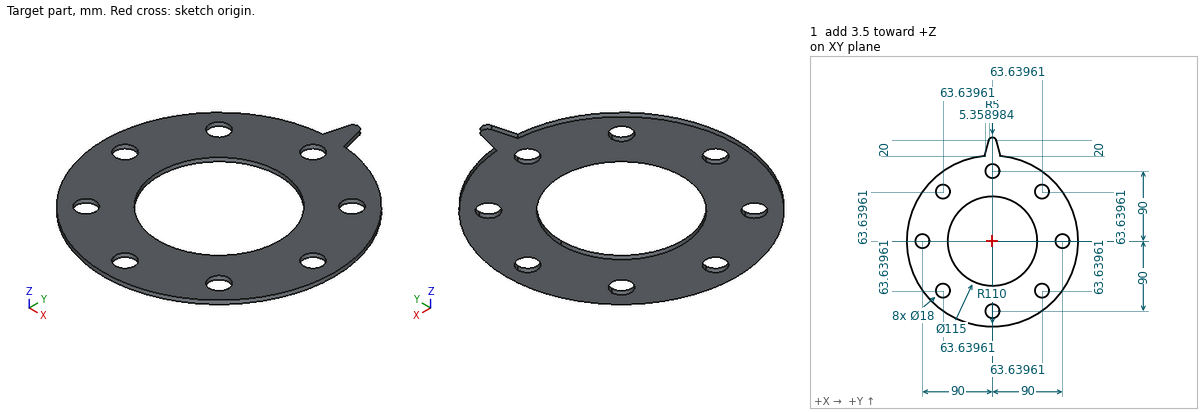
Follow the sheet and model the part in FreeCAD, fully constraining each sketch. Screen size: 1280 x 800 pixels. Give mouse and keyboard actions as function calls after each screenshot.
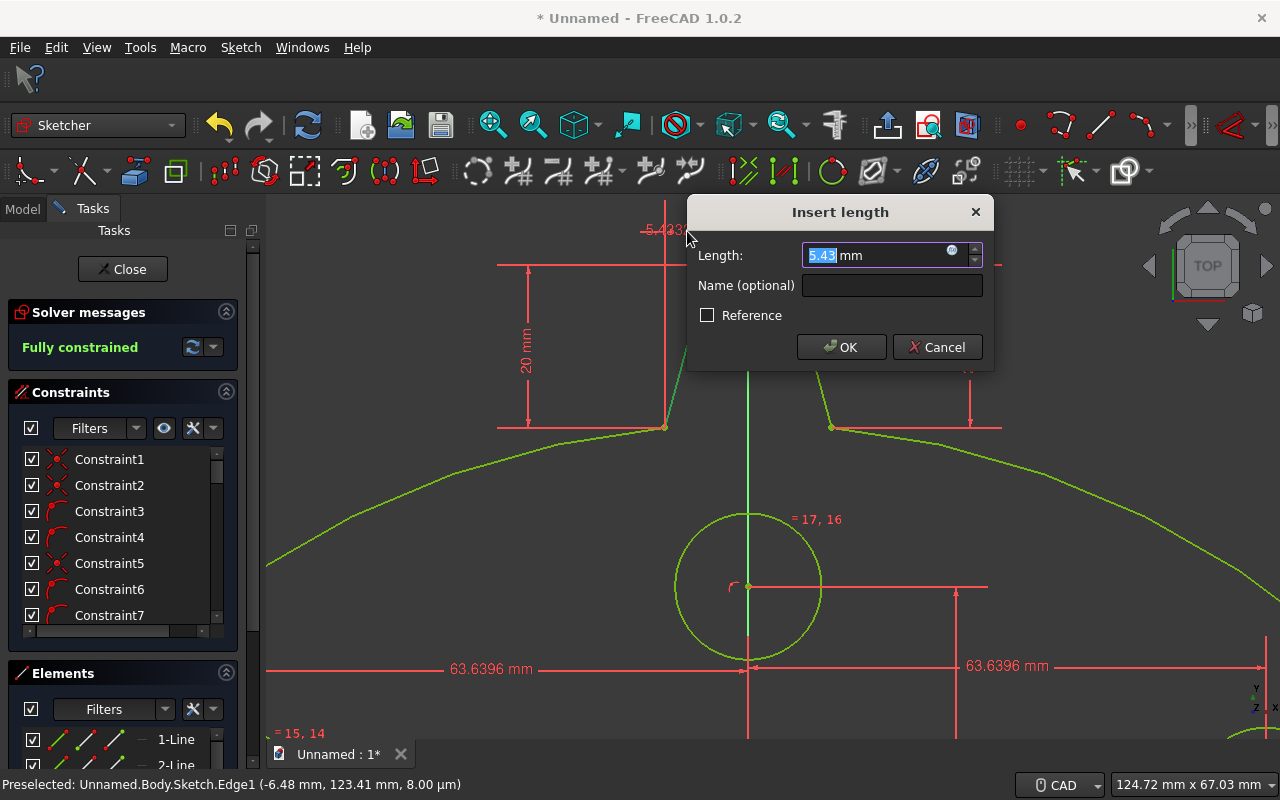
text(5.358984)
key(Return)
key(Escape)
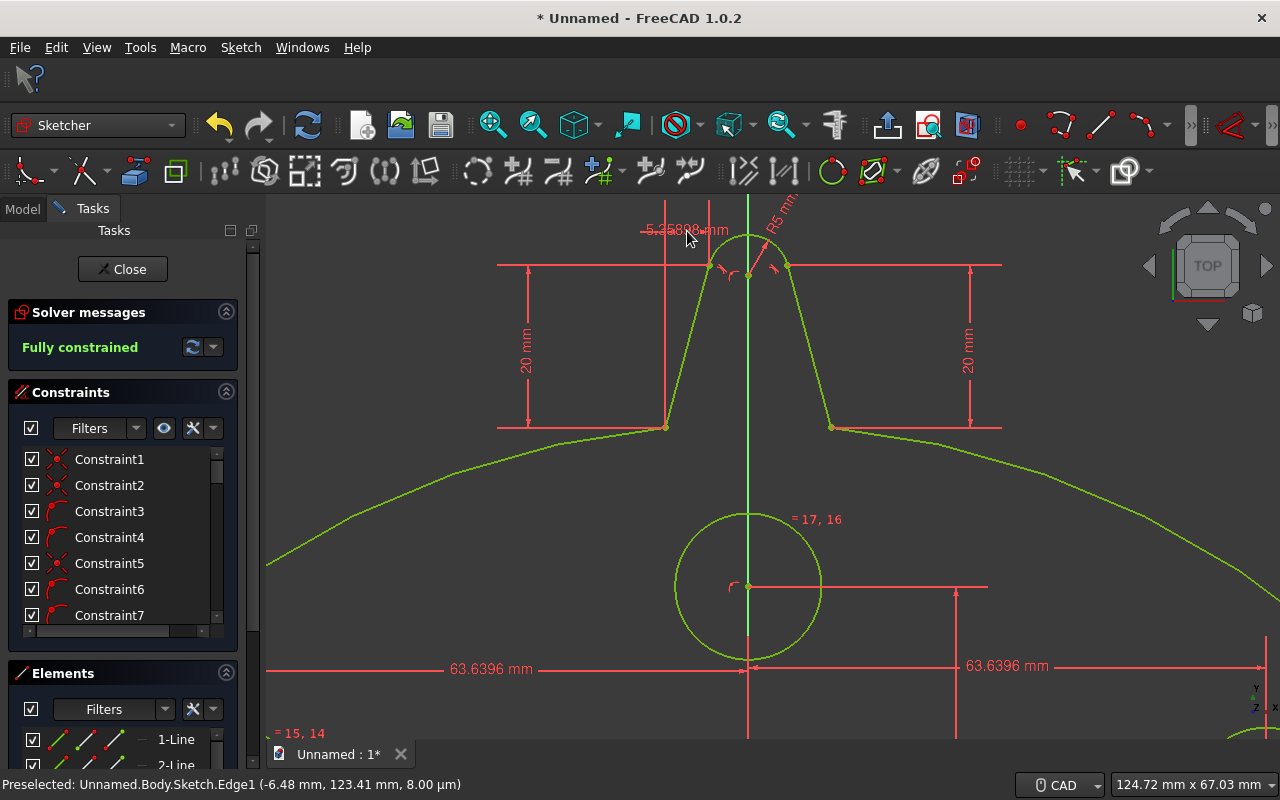
click(123, 269)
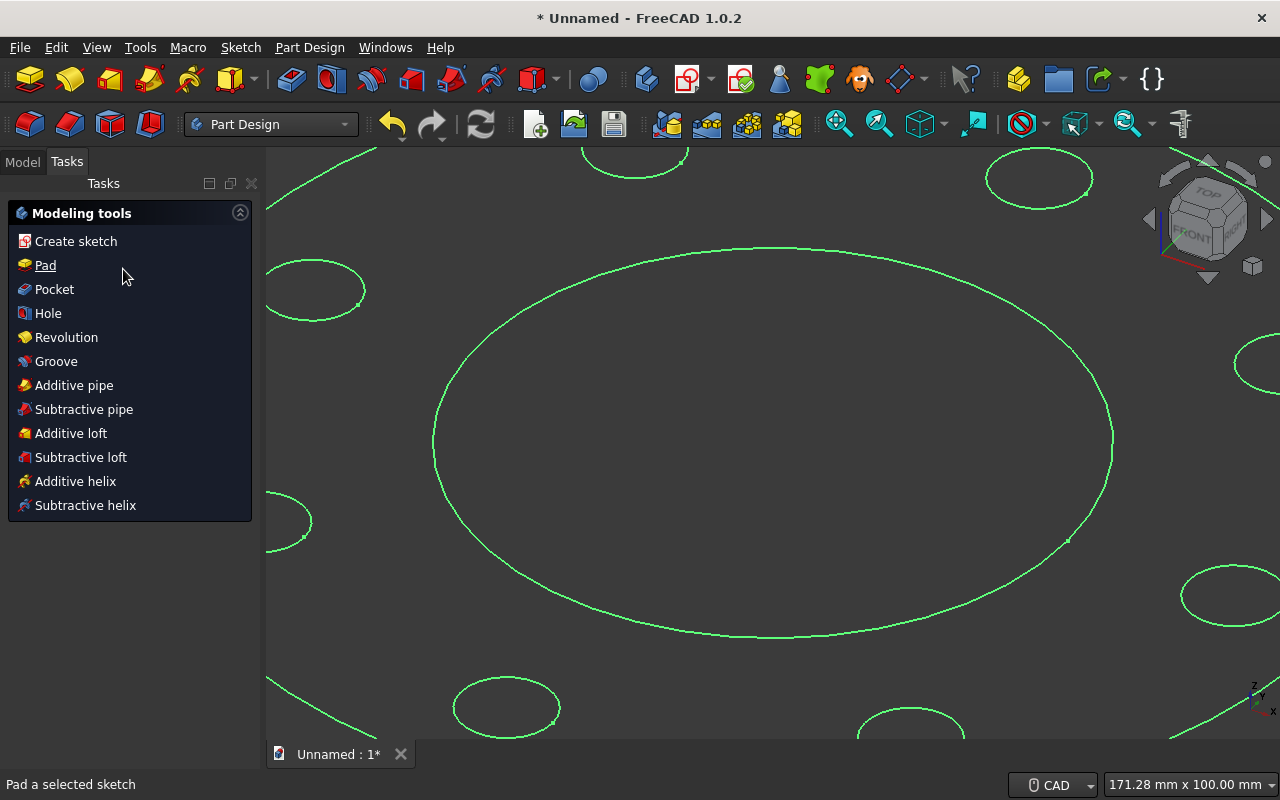
click(30, 80)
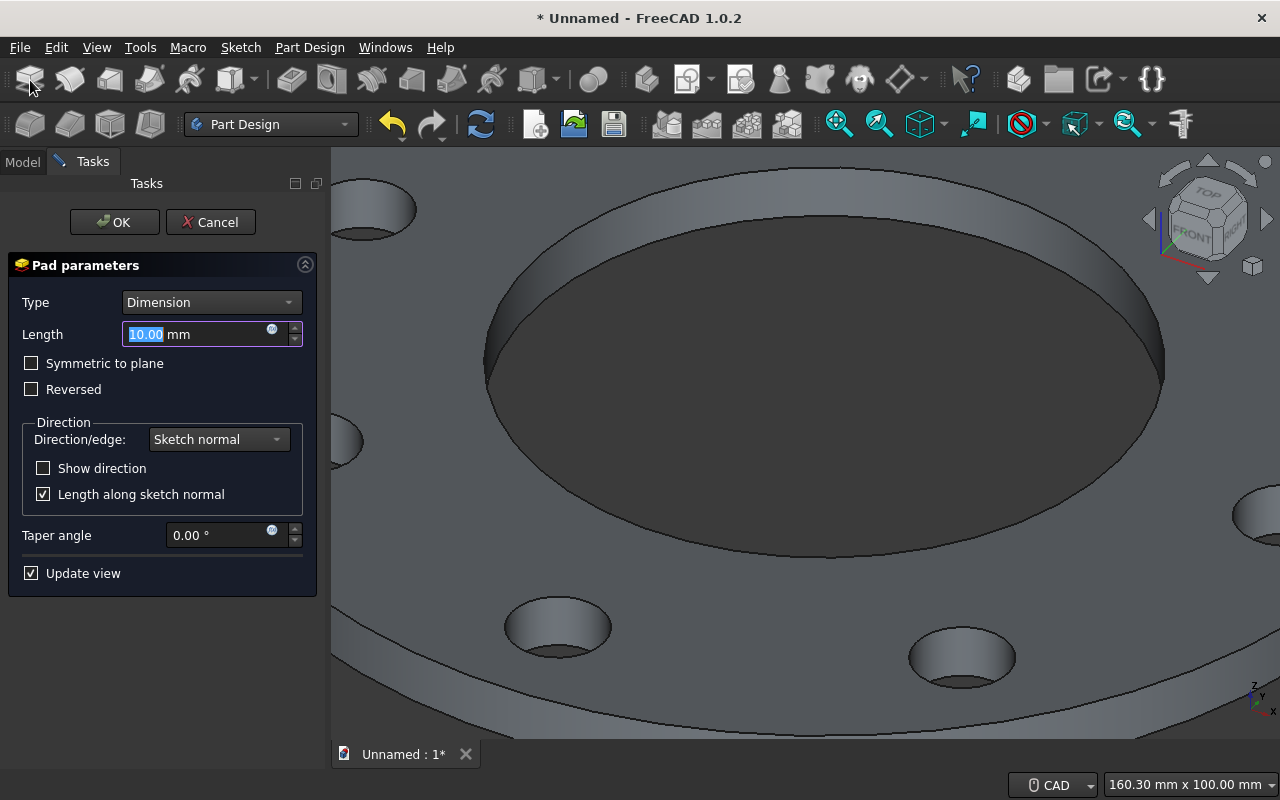
text(3.5)
key(Tab)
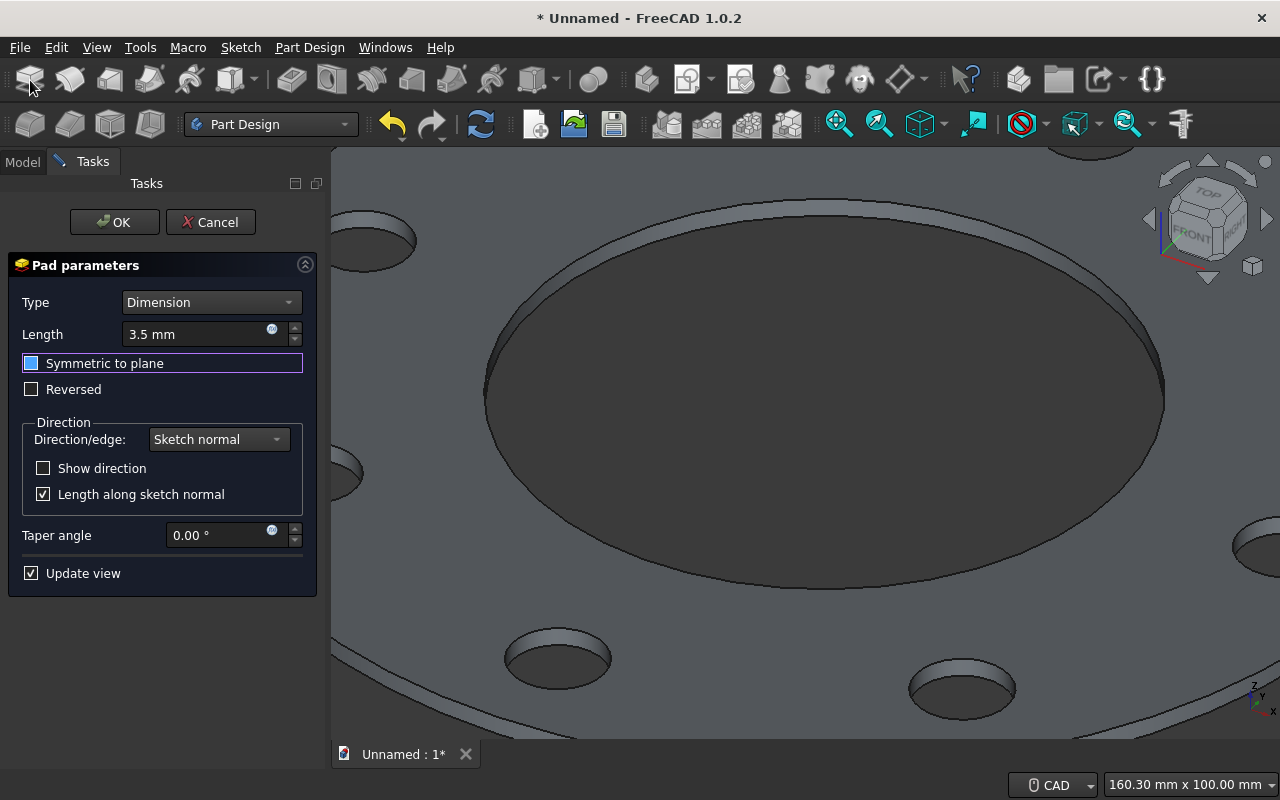
click(115, 222)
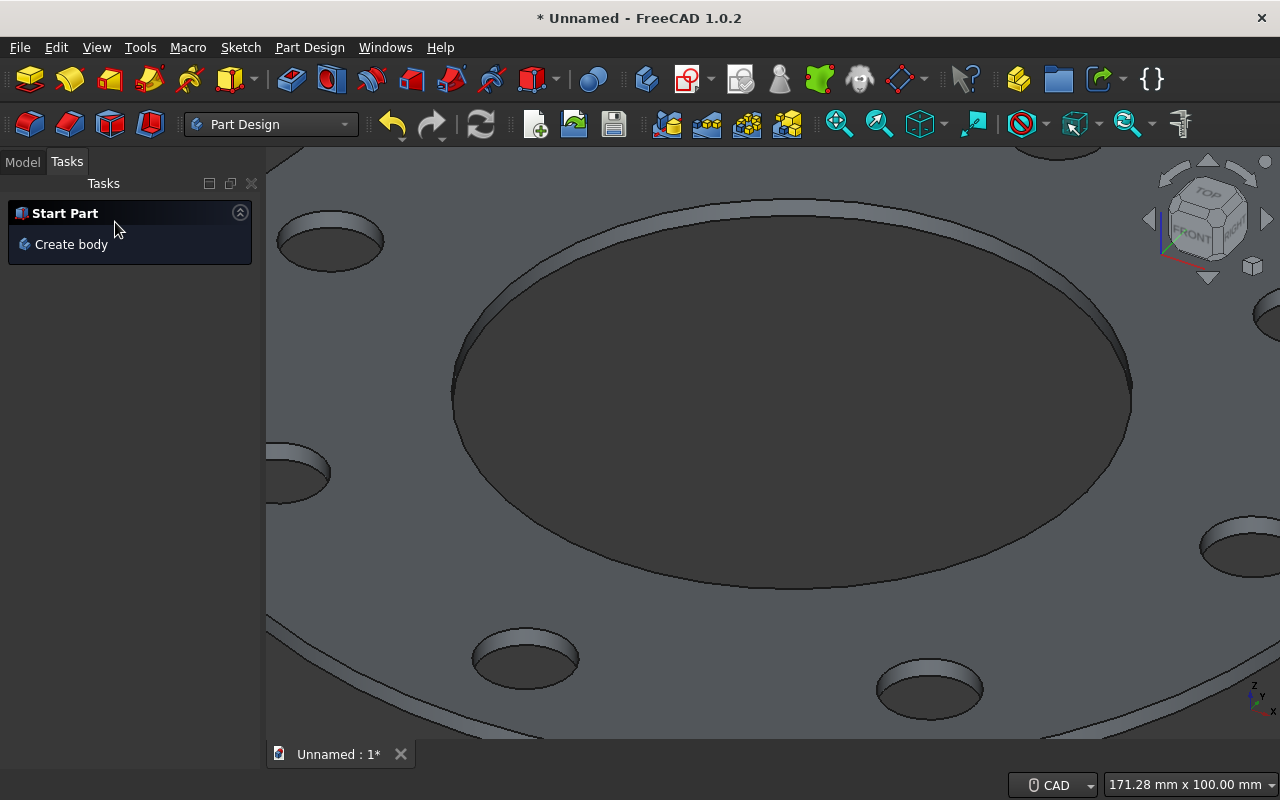
key(0)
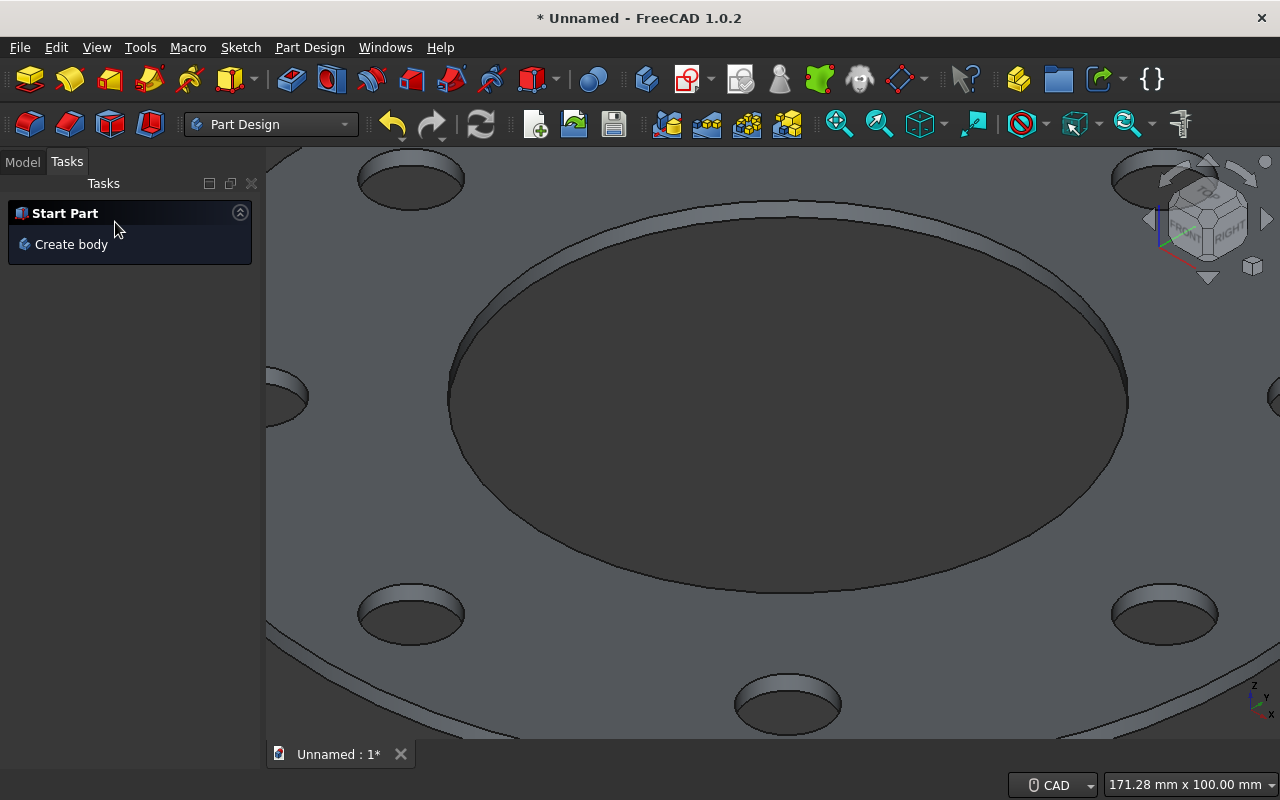
click(840, 124)